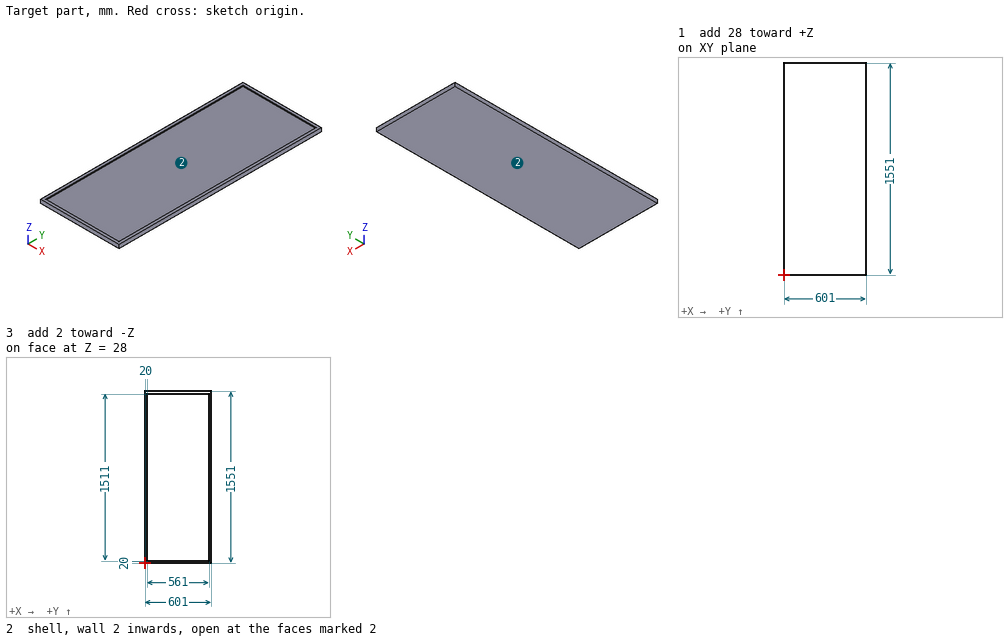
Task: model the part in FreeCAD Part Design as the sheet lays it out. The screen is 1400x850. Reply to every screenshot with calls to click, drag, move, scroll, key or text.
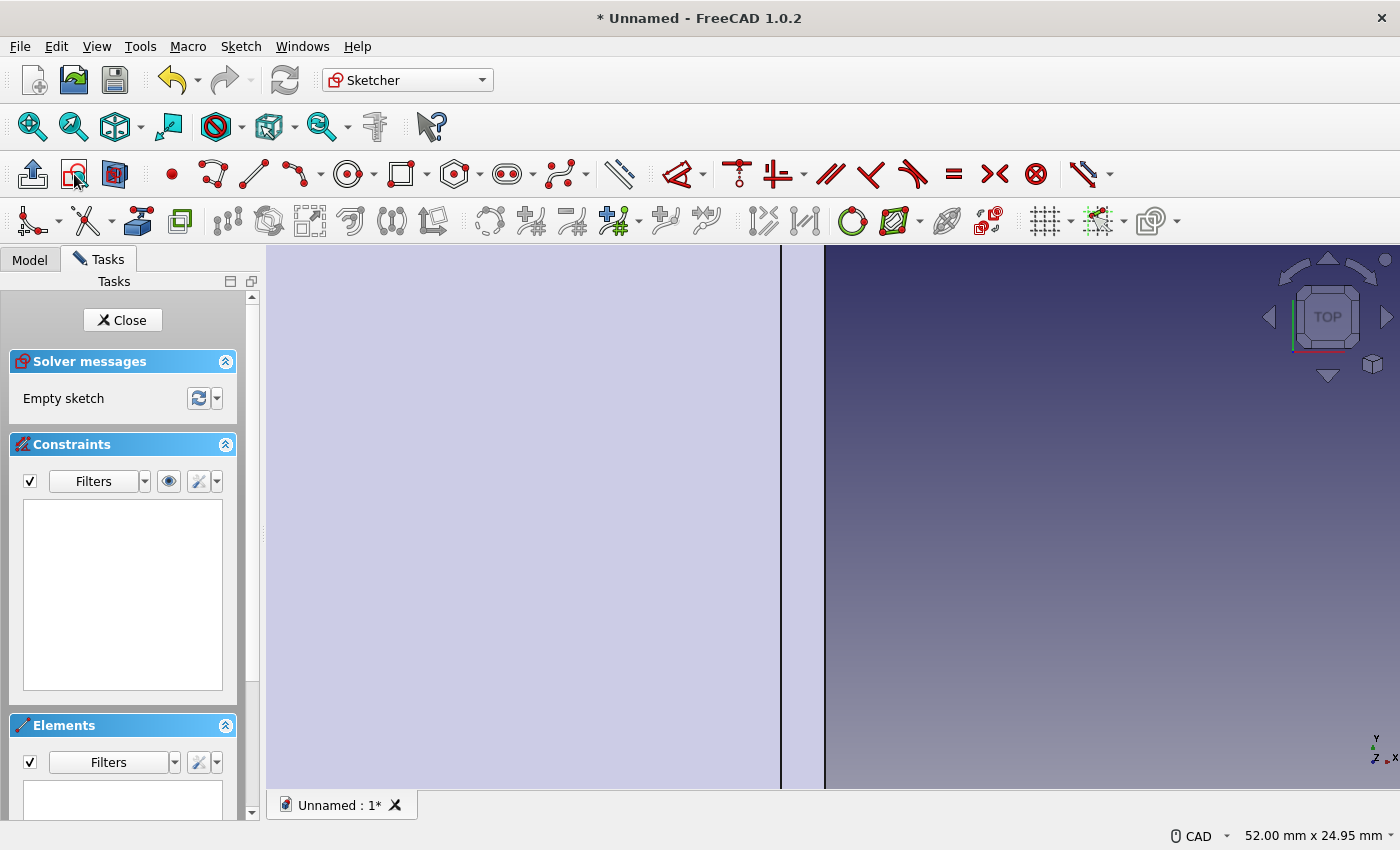
scroll(764, 517, down, 15)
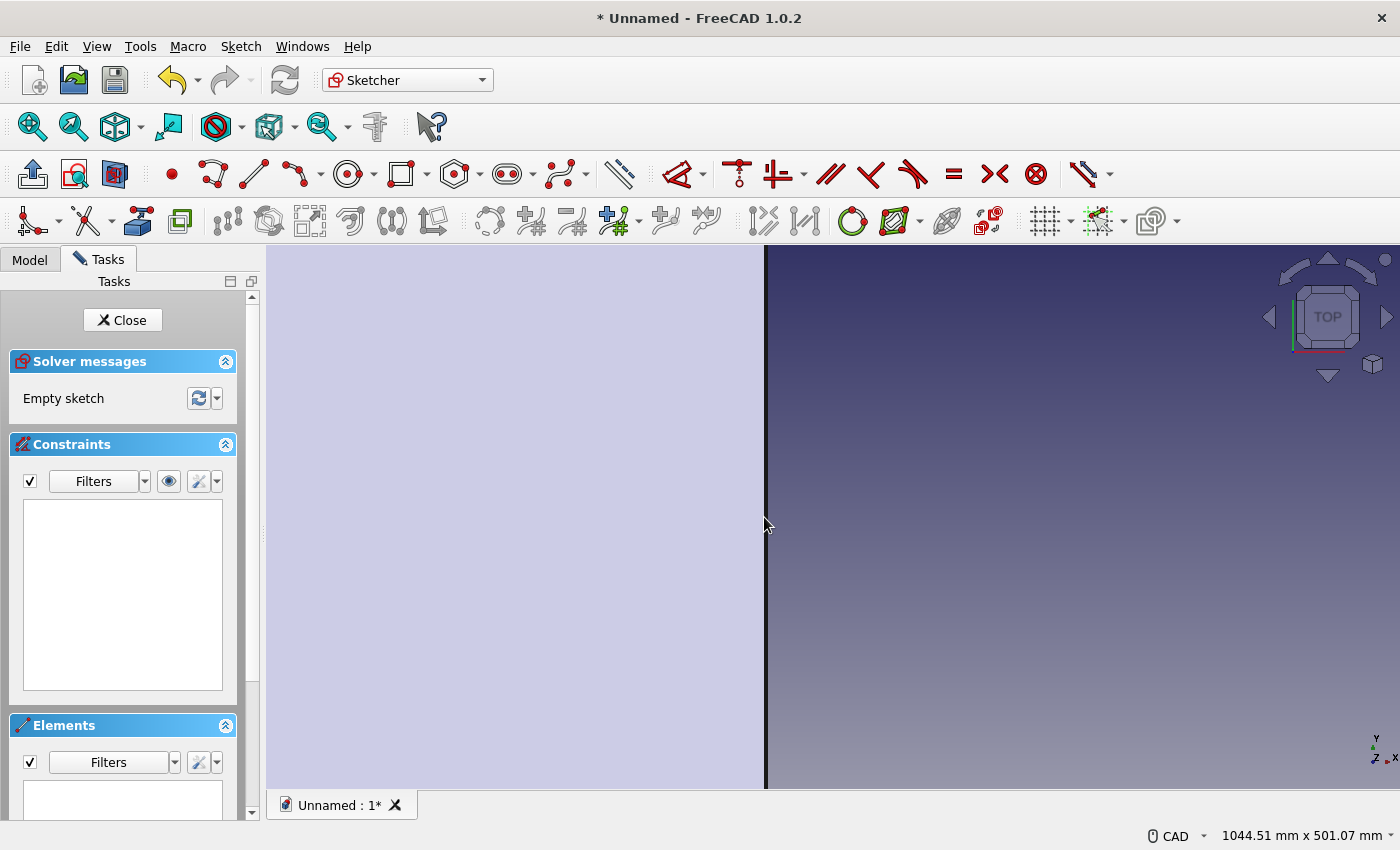
scroll(846, 403, down, 8)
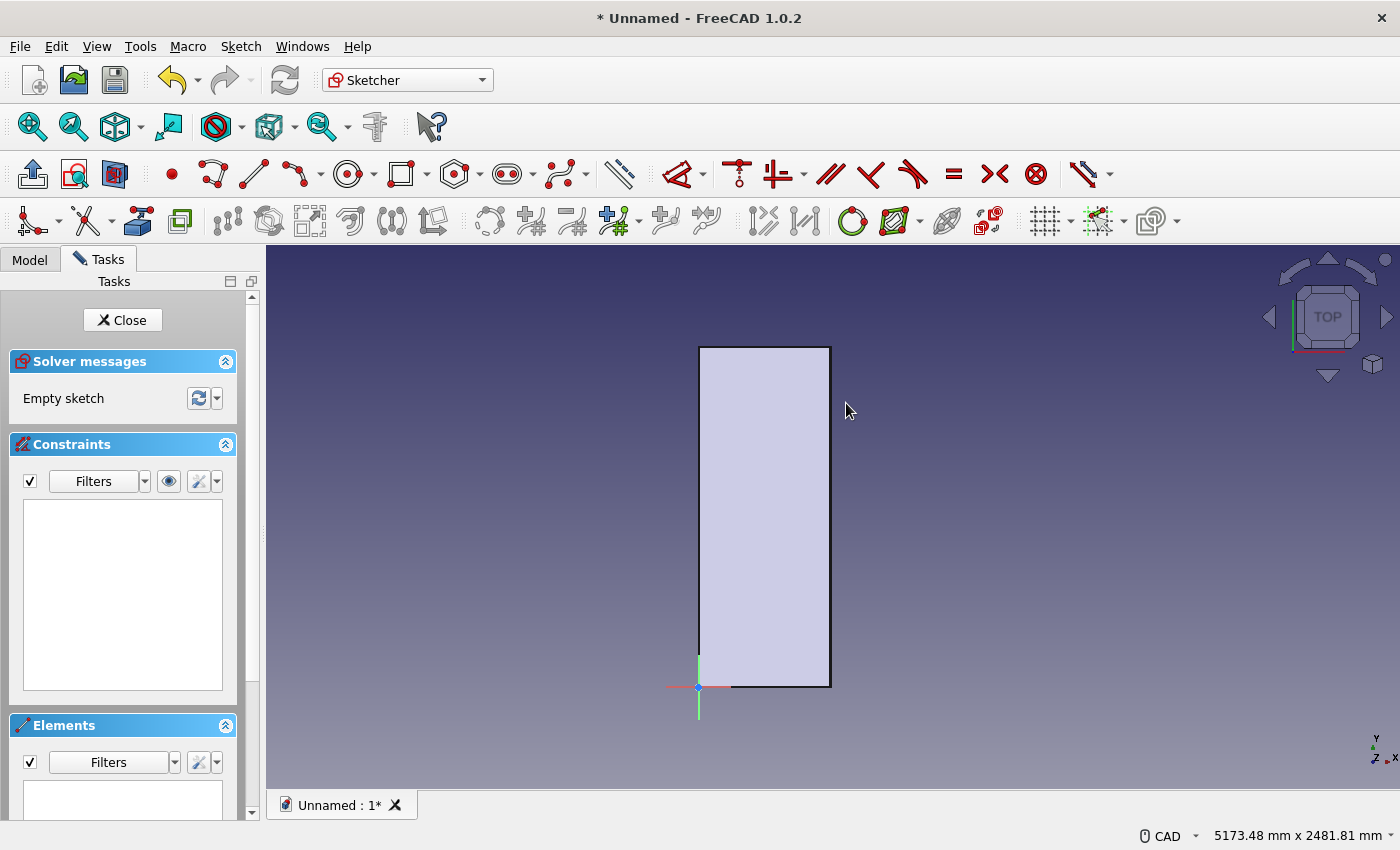
click(400, 174)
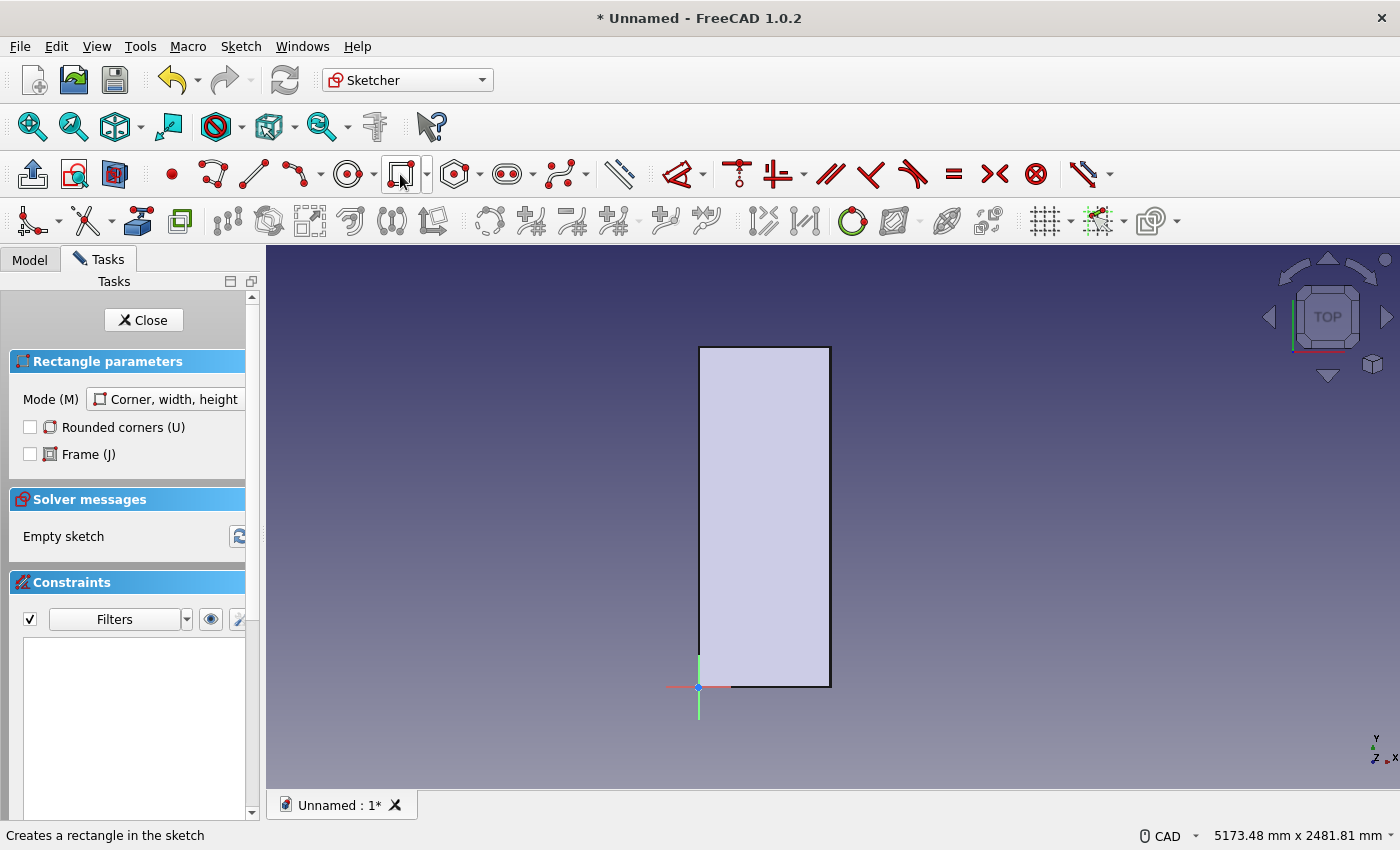
click(699, 687)
click(831, 347)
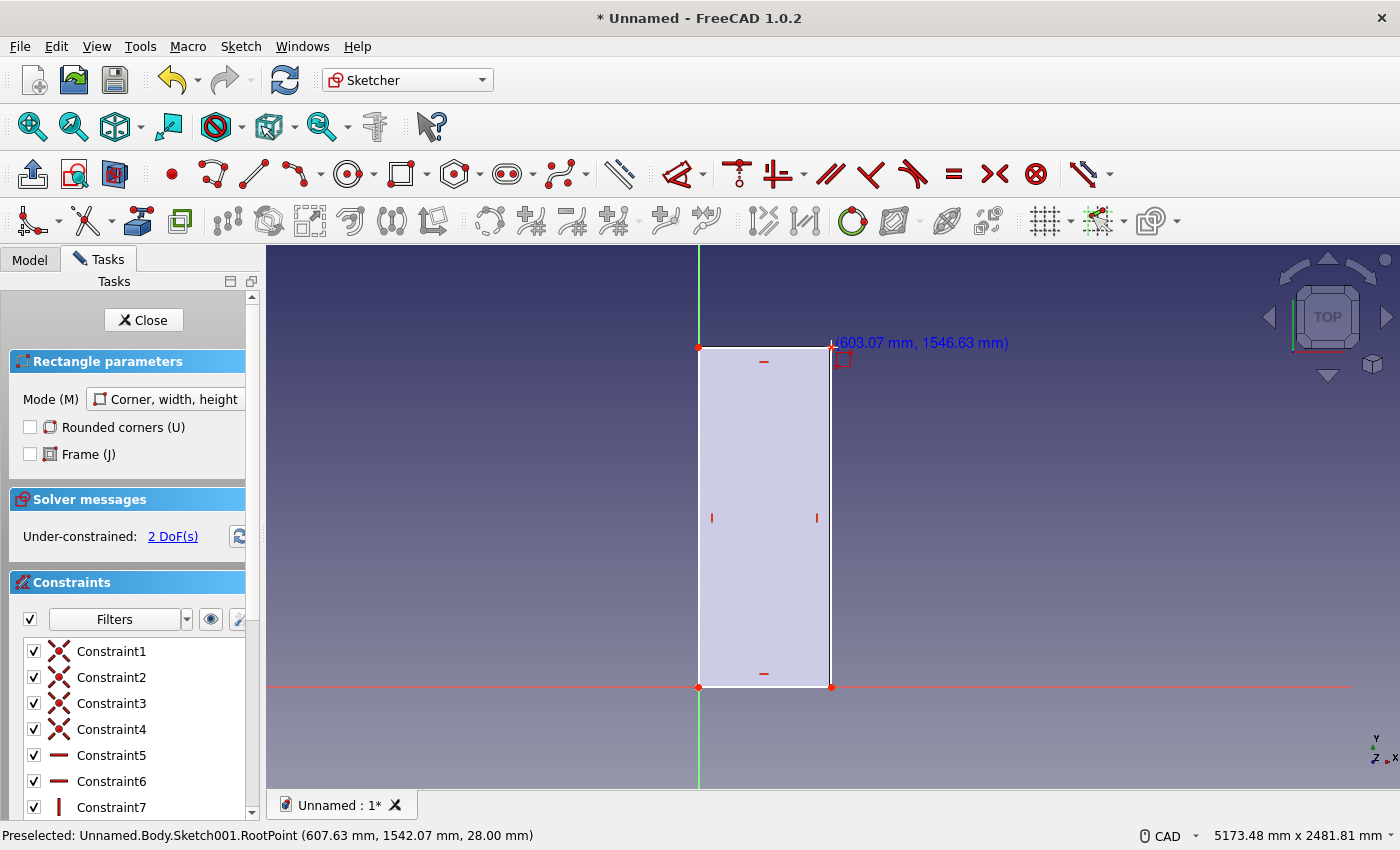
scroll(703, 351, up, 7)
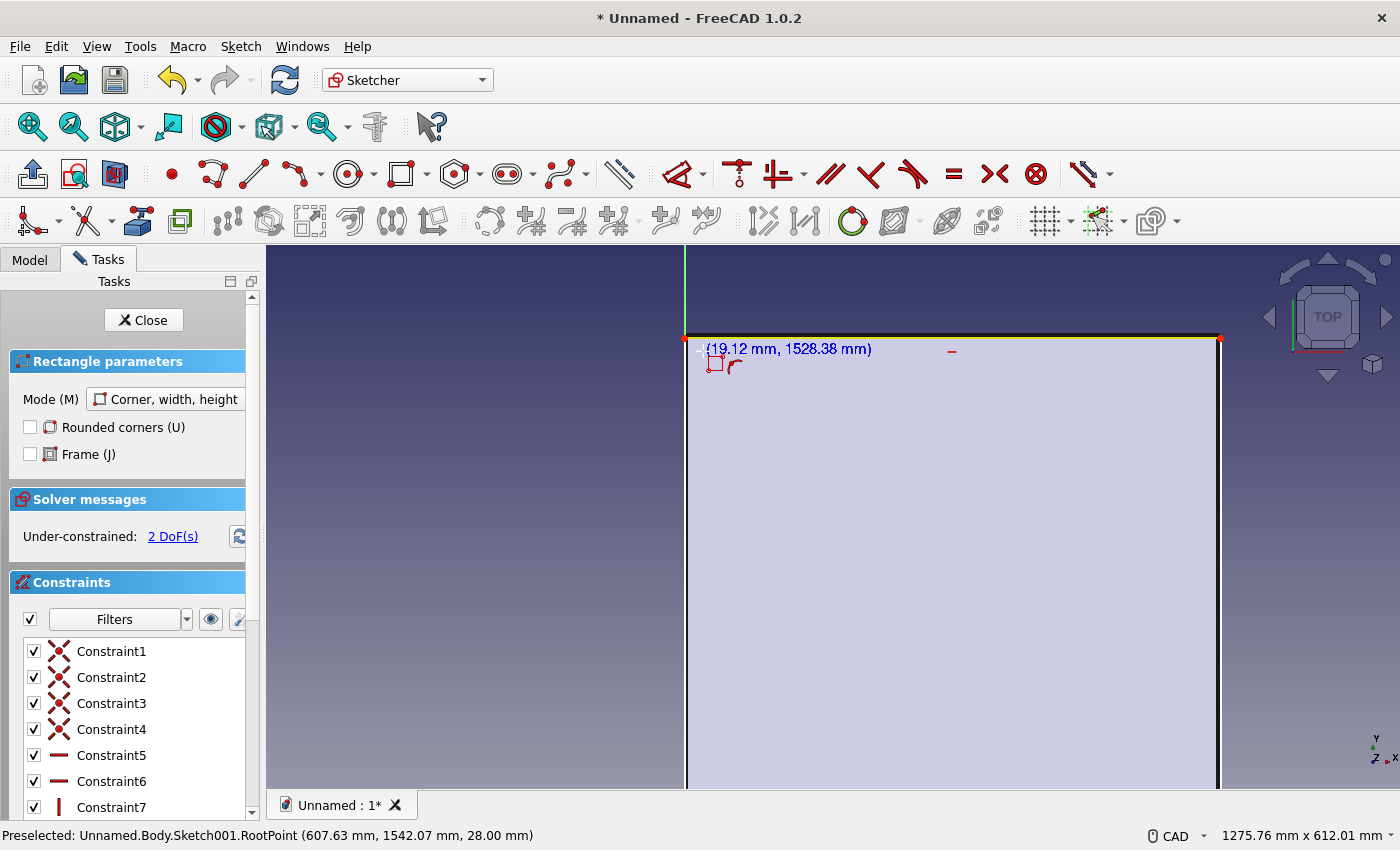
click(703, 352)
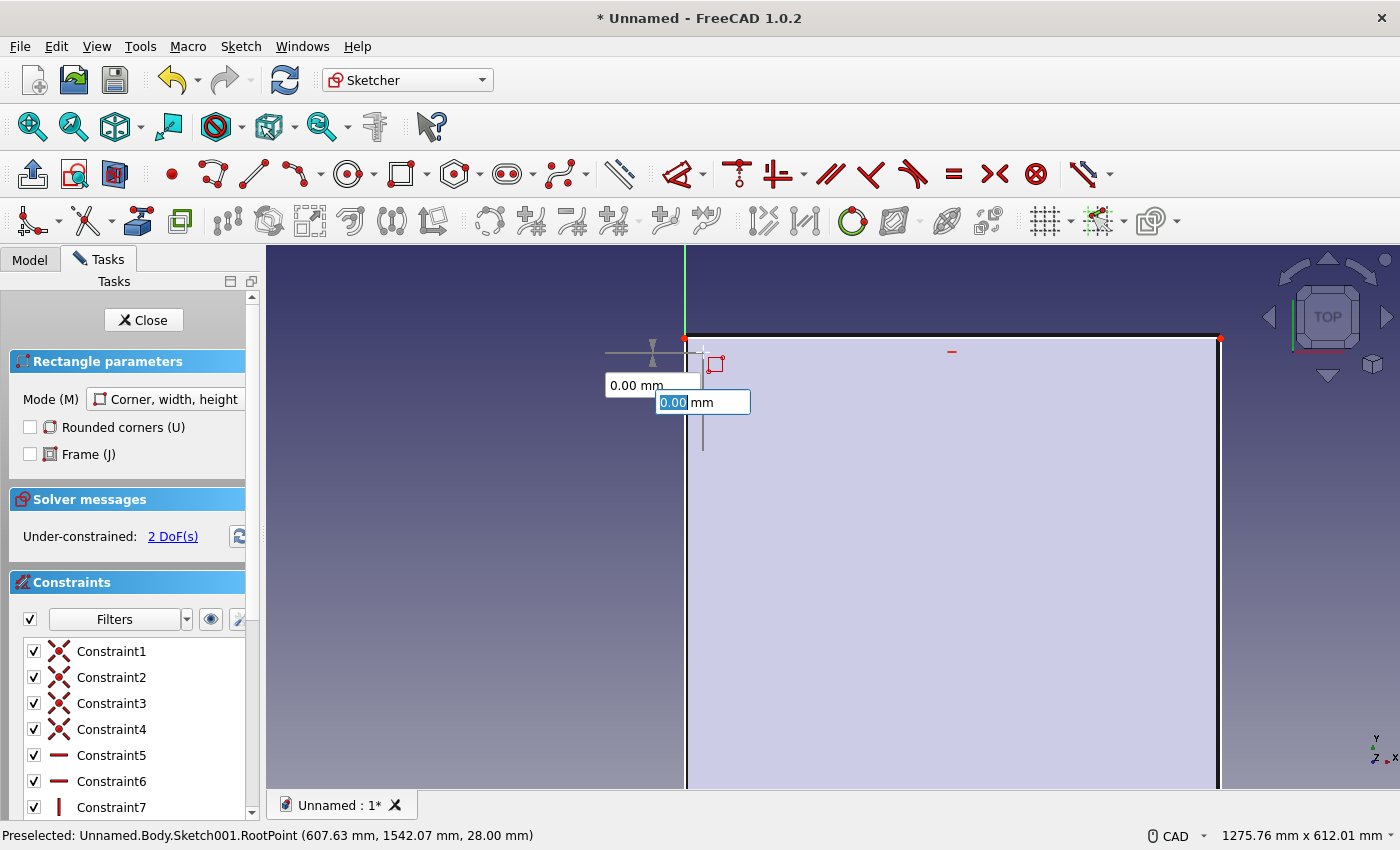
scroll(703, 351, down, 7)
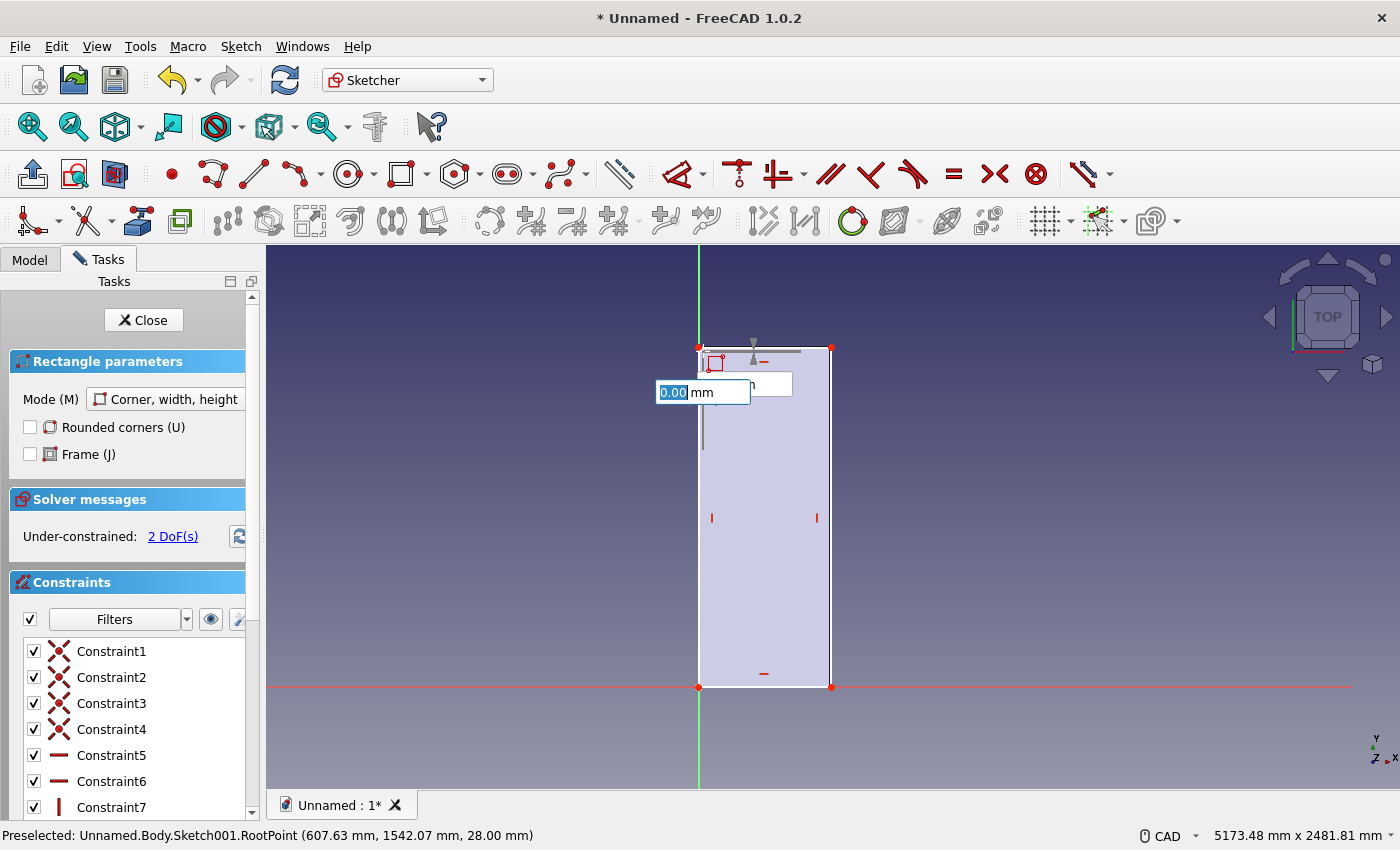
scroll(826, 683, up, 7)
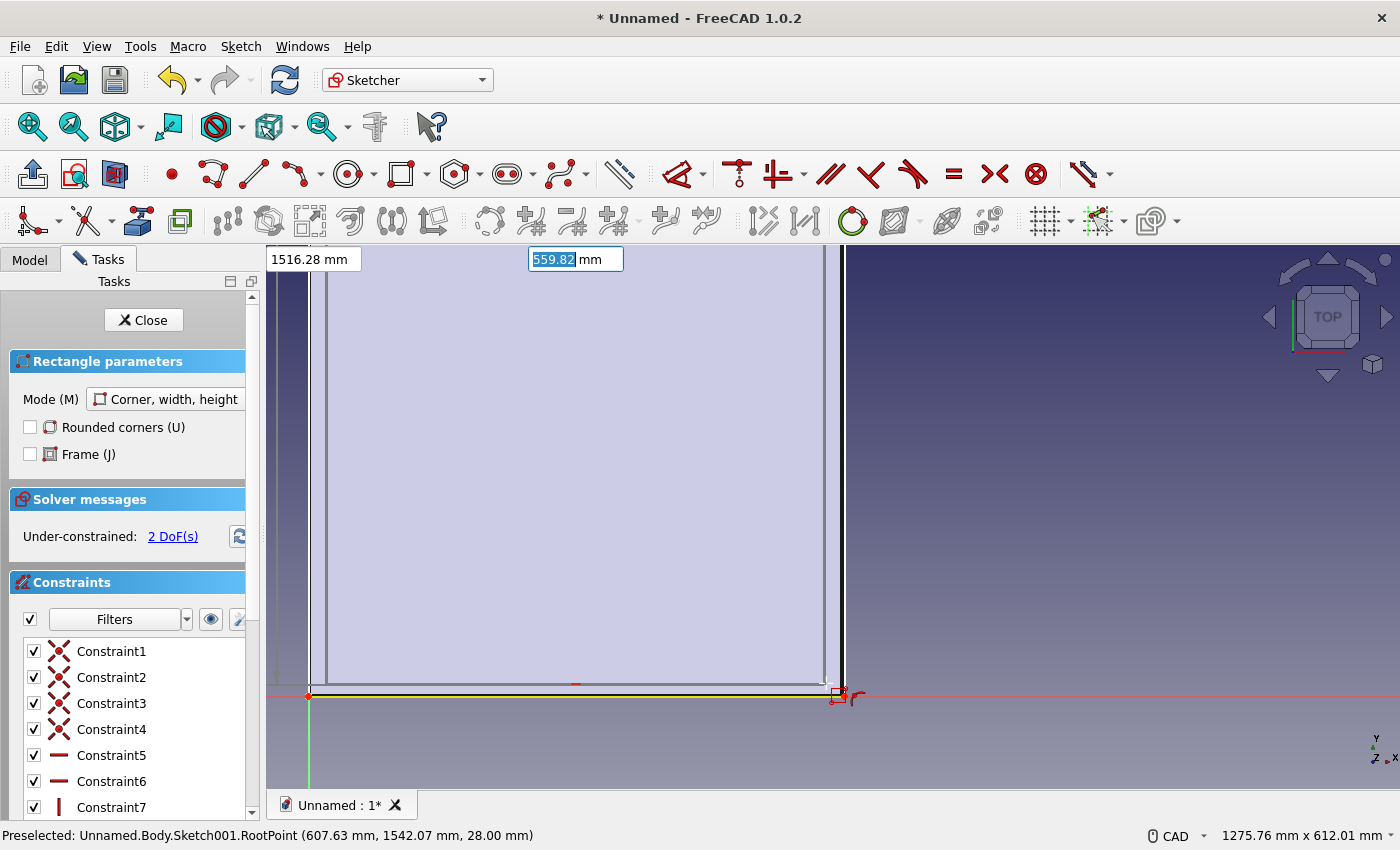
click(825, 679)
key(Escape)